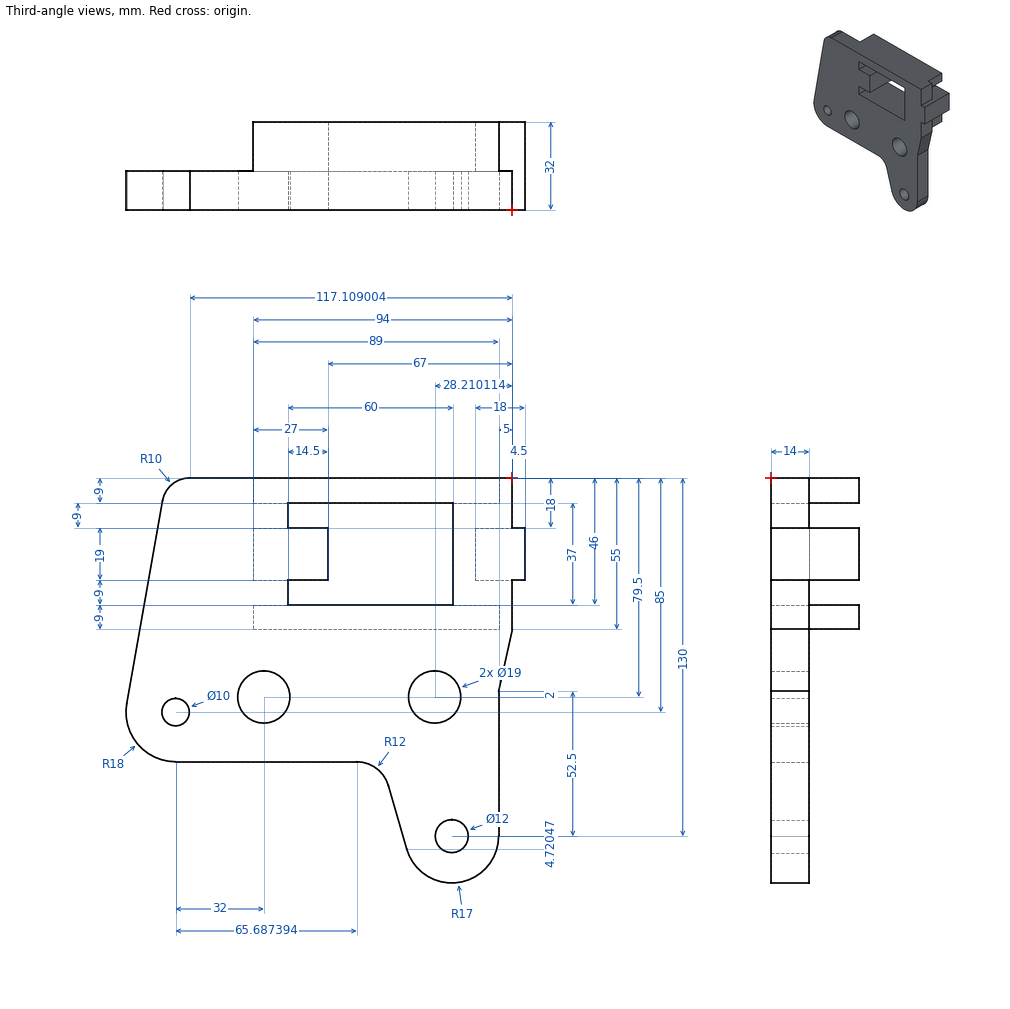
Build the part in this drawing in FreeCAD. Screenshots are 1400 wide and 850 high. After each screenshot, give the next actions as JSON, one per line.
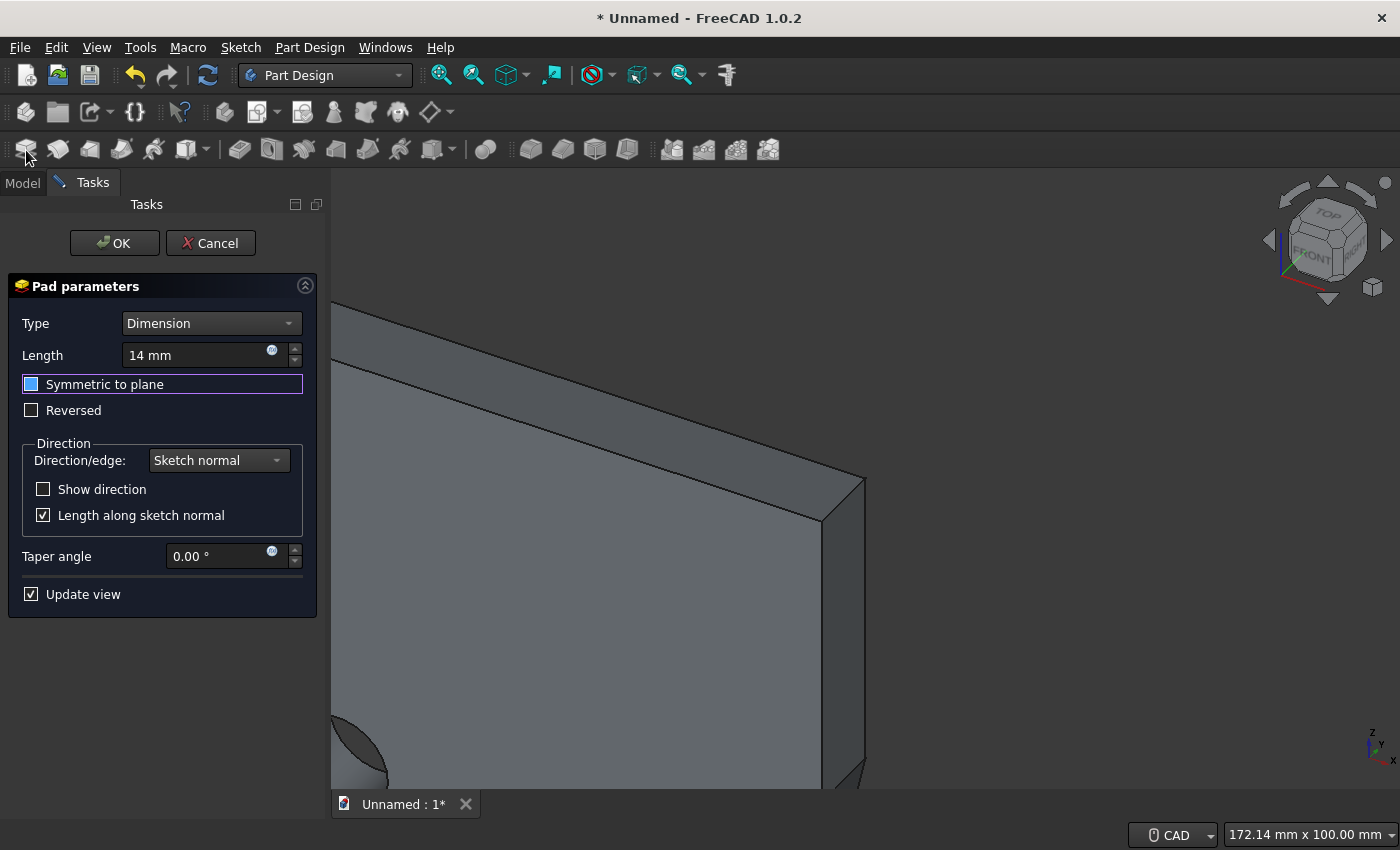
{"action": "left_click", "coordinate": [30, 410]}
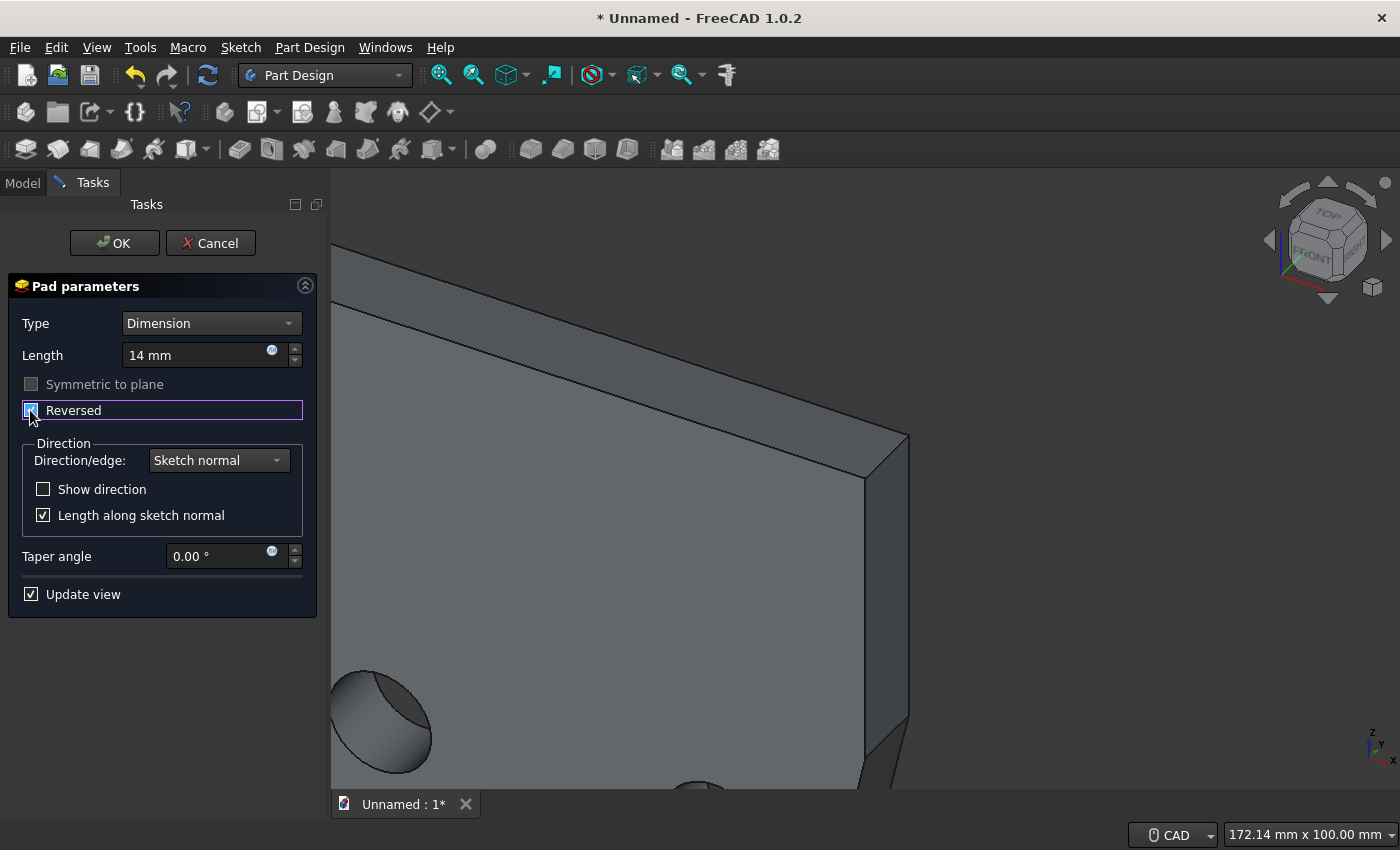
{"action": "left_click", "coordinate": [115, 243]}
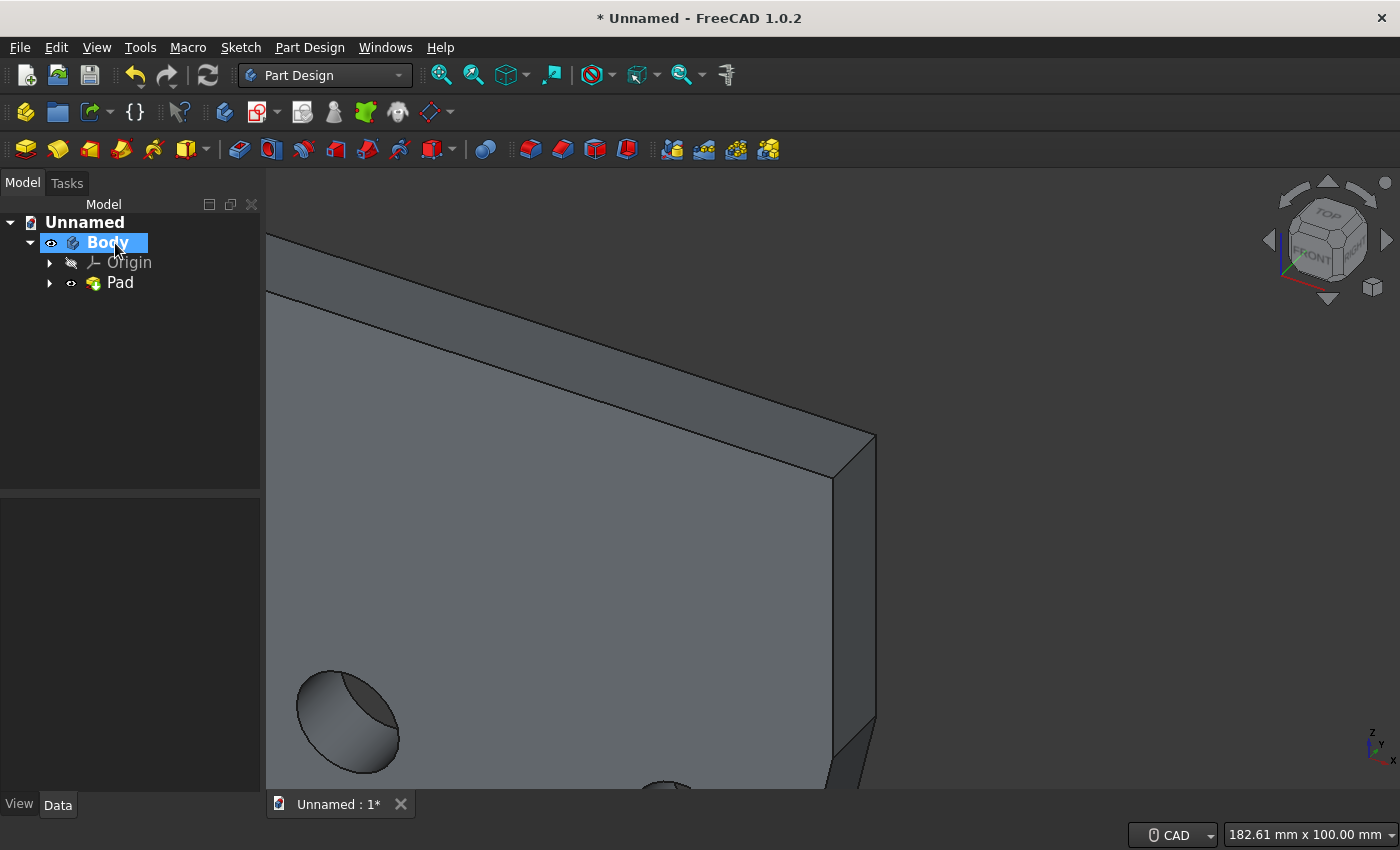
{"action": "left_click", "coordinate": [442, 76]}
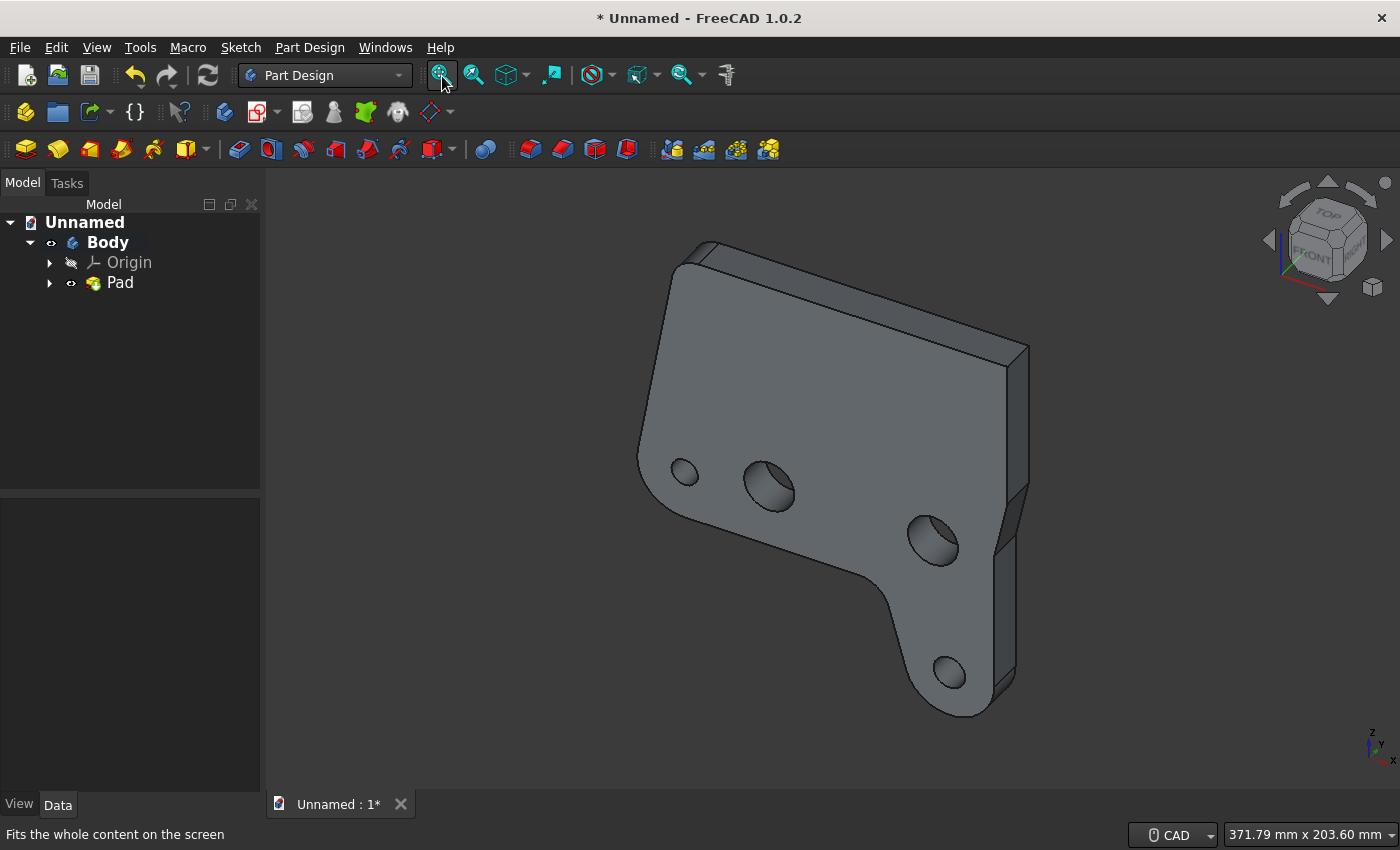
{"action": "left_click", "coordinate": [258, 112]}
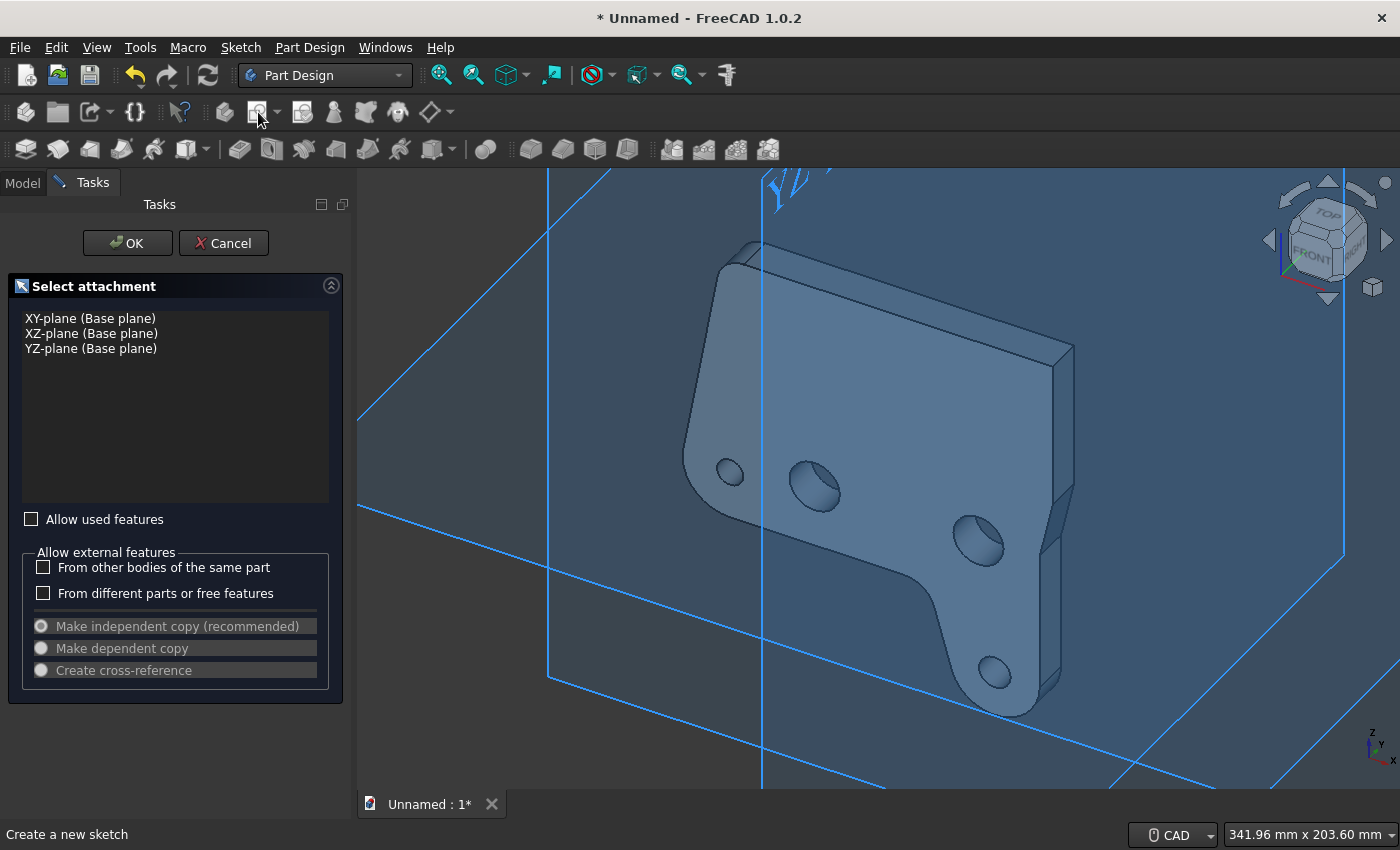
{"action": "left_click", "coordinate": [82, 334]}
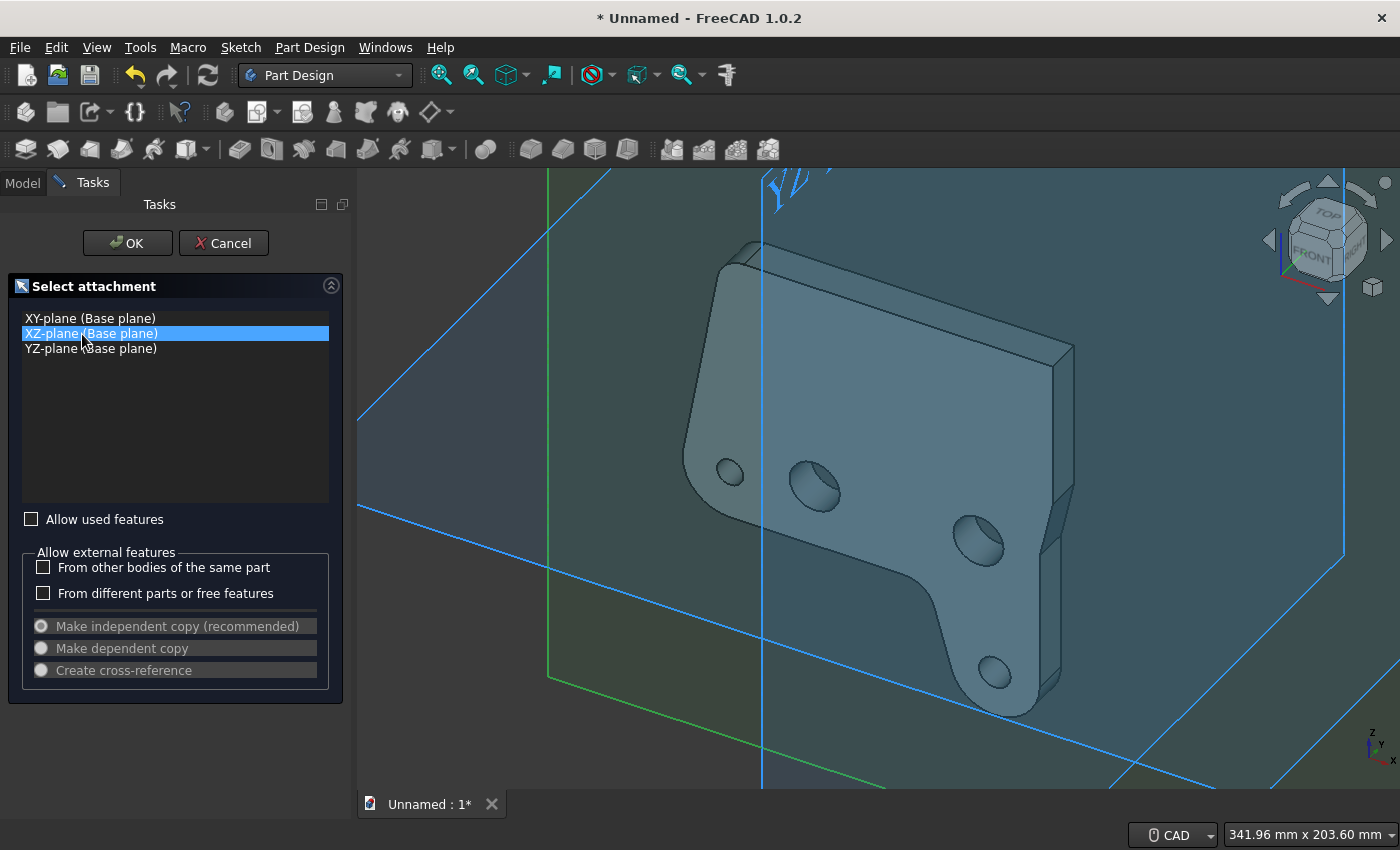
{"action": "left_click", "coordinate": [128, 243]}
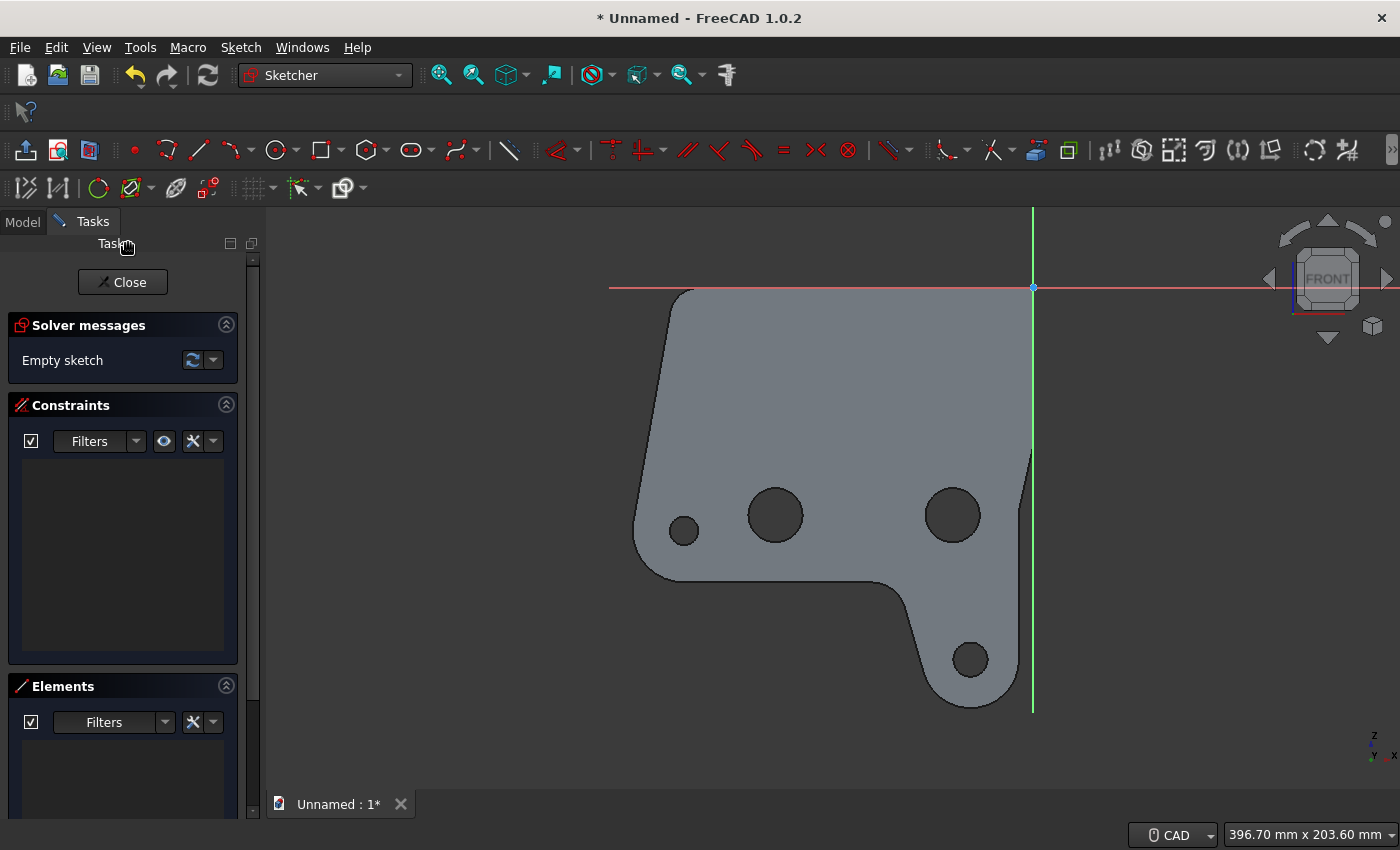
{"action": "scroll", "coordinate": [1021, 259], "scroll_direction": "up", "scroll_amount": 4}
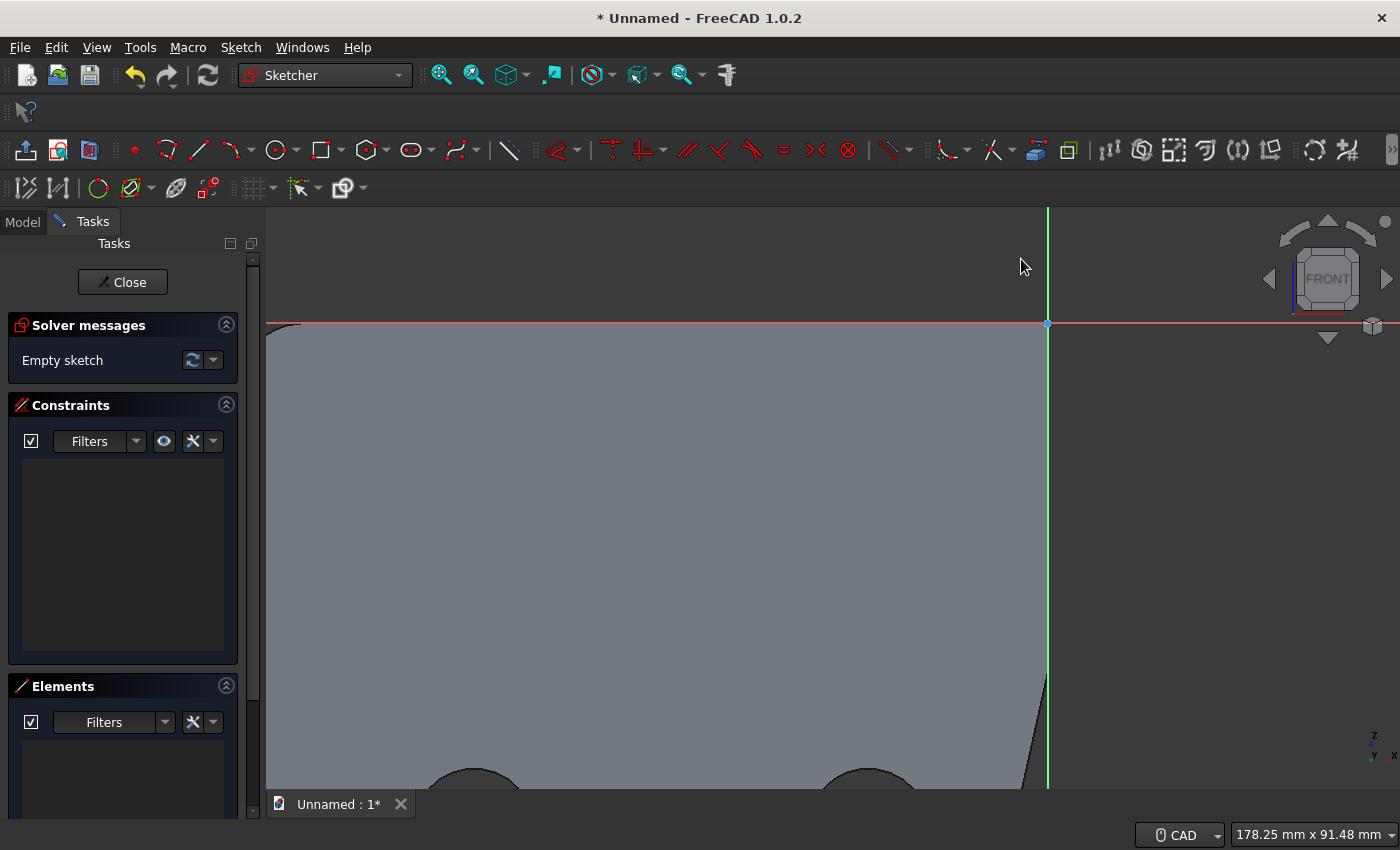
{"action": "left_click", "coordinate": [322, 150]}